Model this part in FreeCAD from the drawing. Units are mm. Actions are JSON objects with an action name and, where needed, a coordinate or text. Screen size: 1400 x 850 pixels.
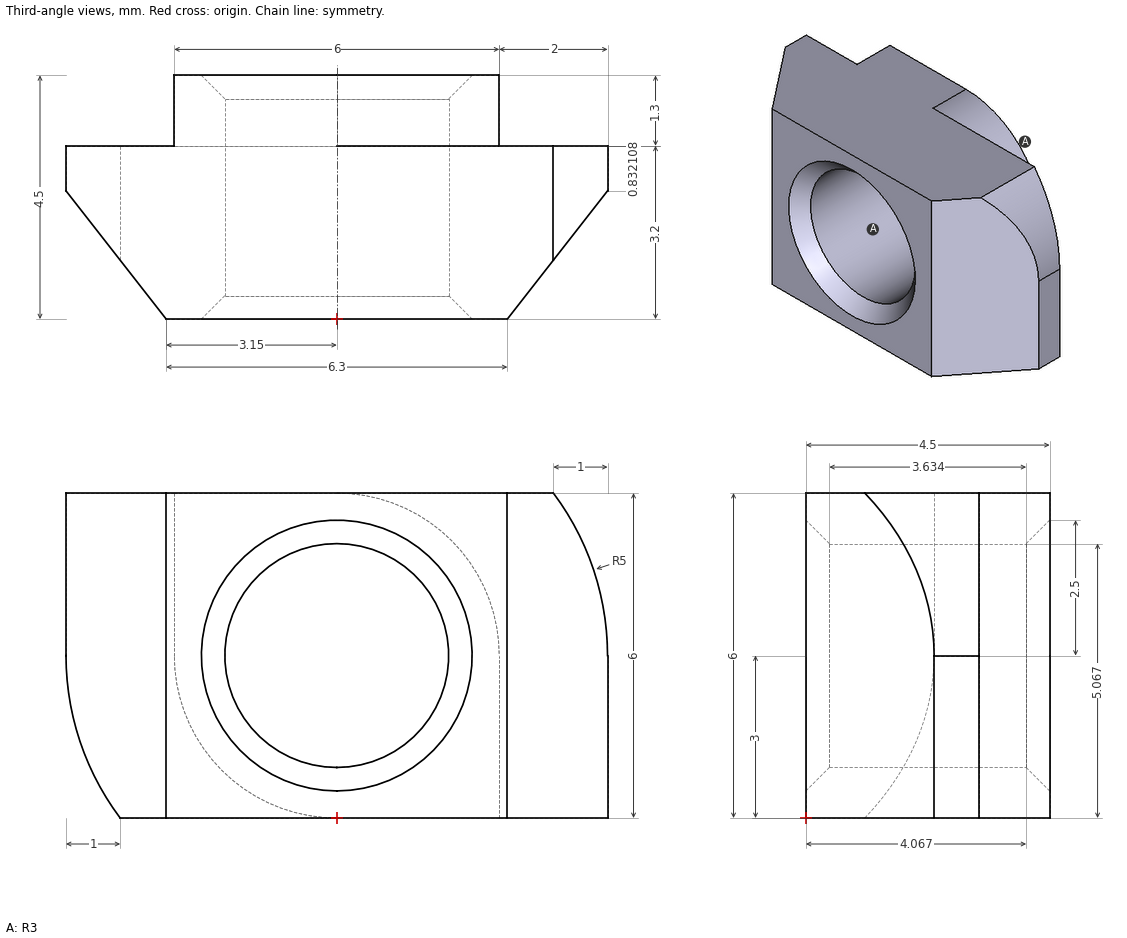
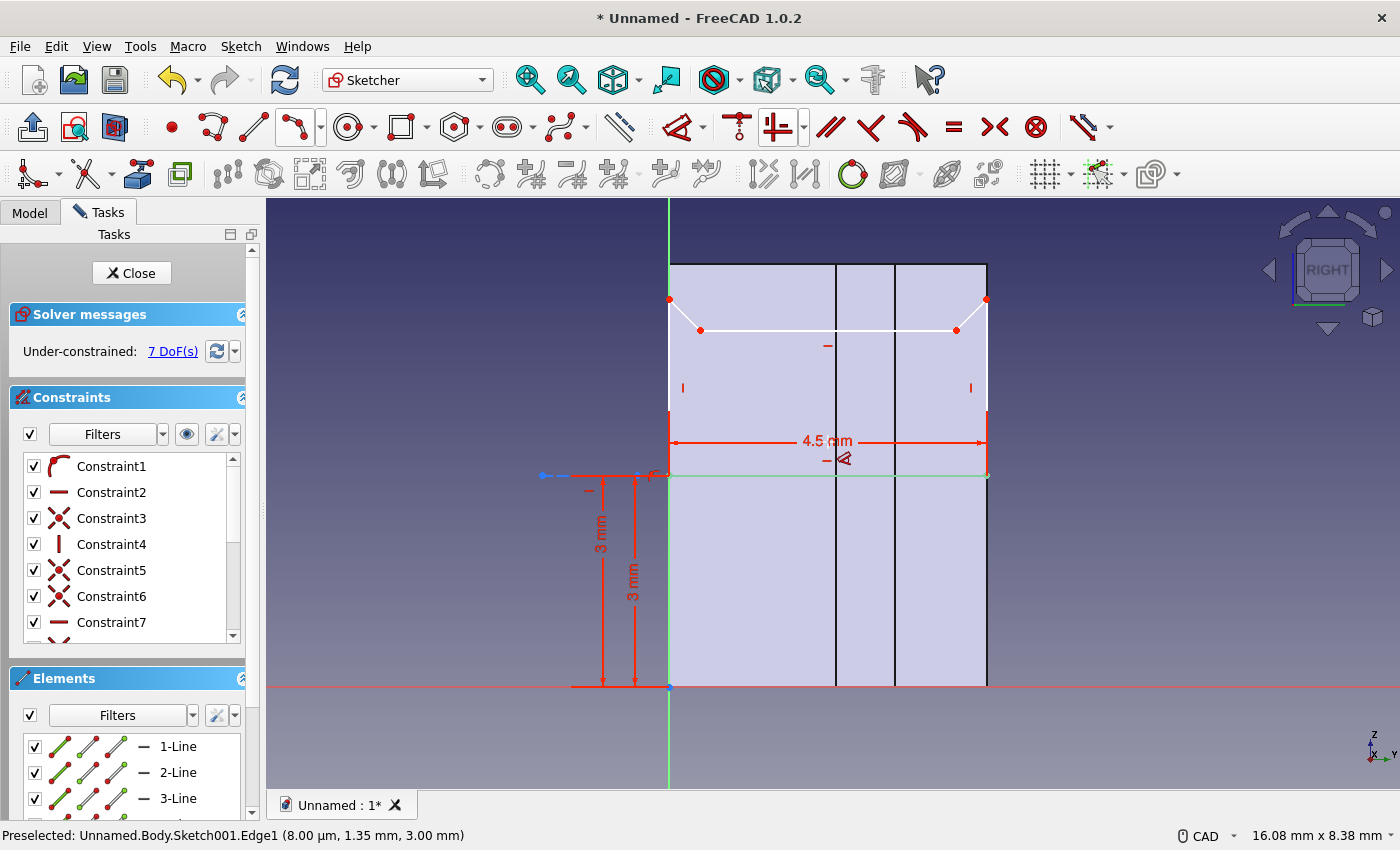
{"action": "left_click", "coordinate": [987, 423]}
{"action": "left_click", "coordinate": [1021, 388]}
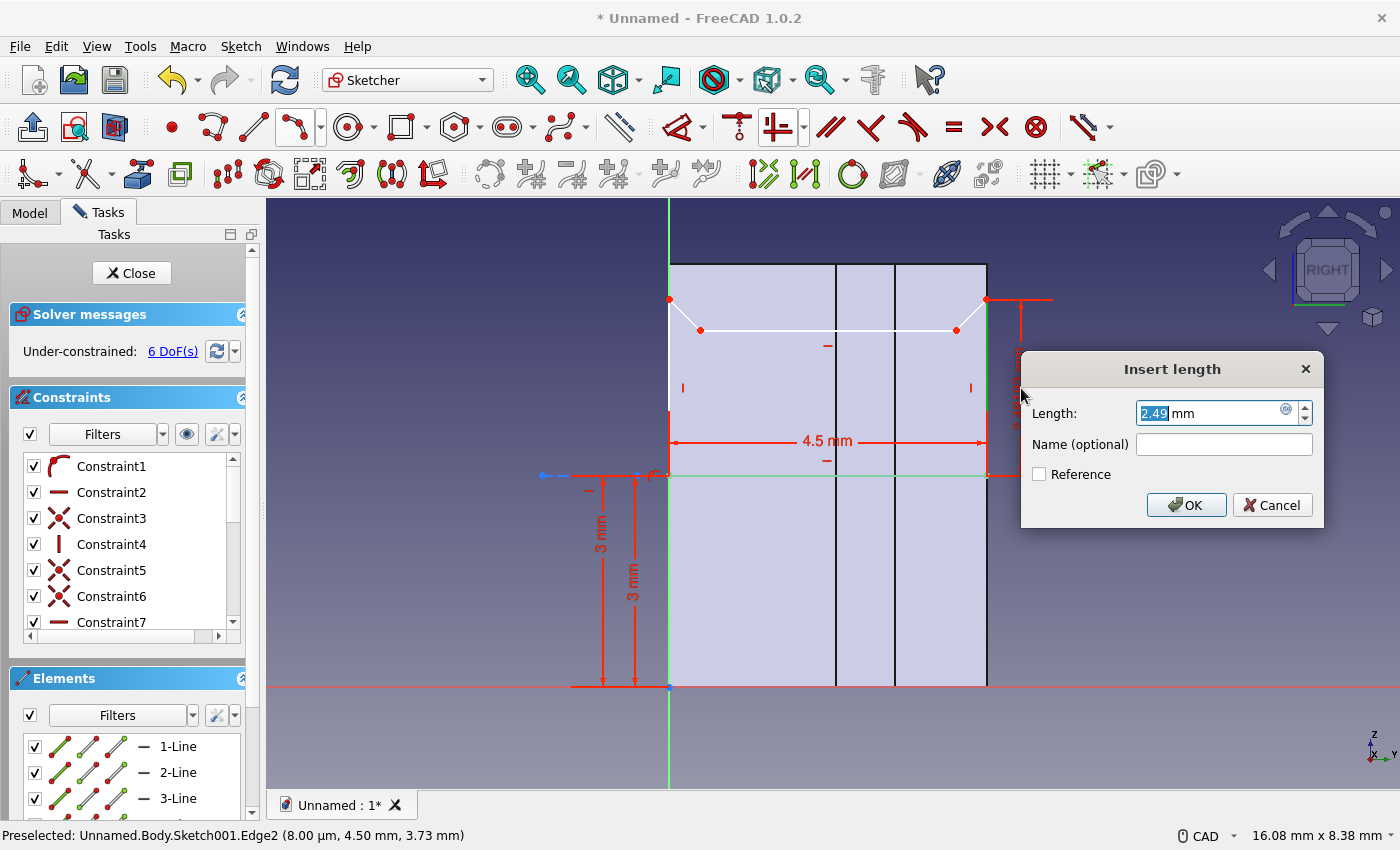
{"action": "type", "text": "2.5"}
{"action": "key", "text": "Return"}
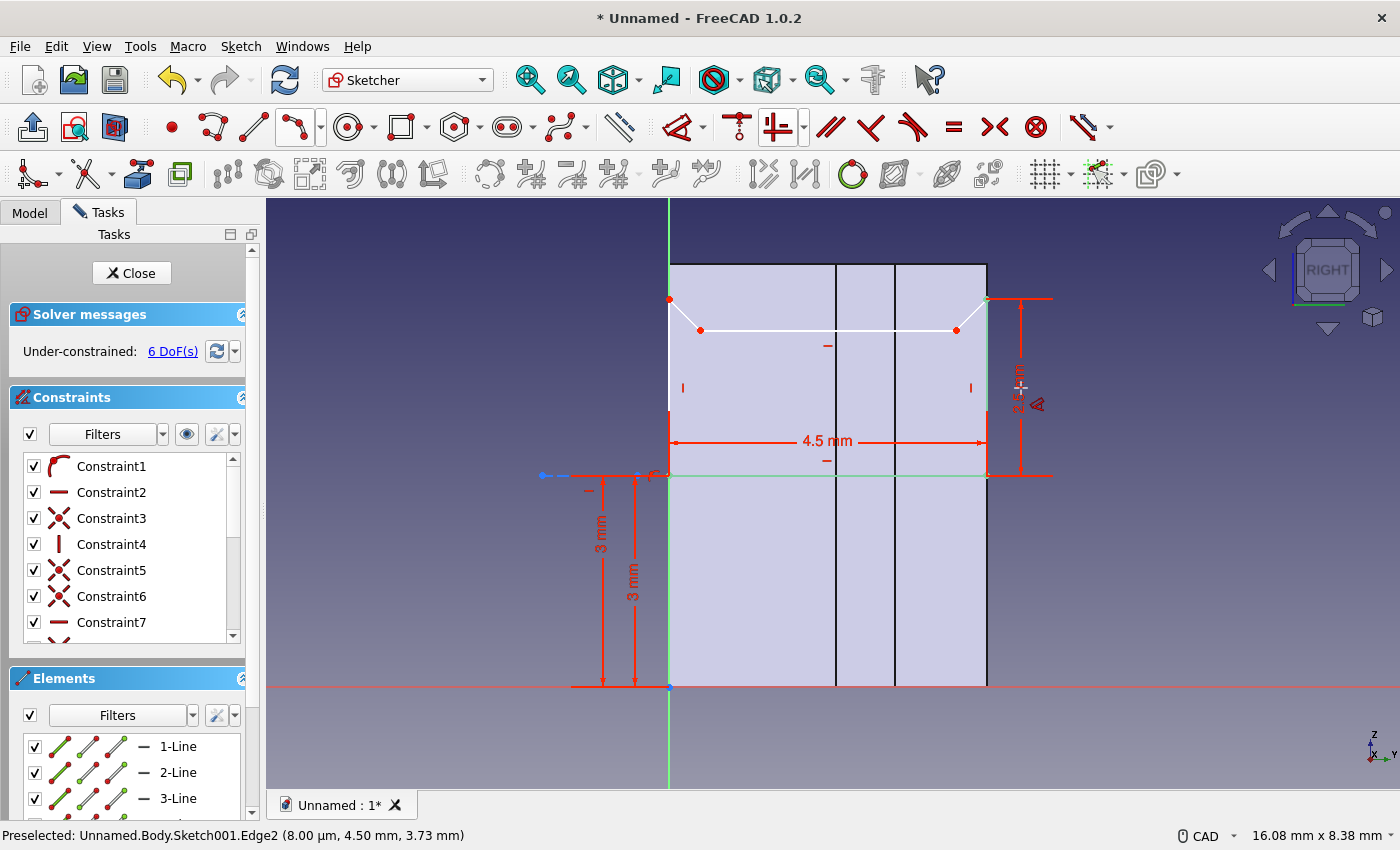
{"action": "left_click", "coordinate": [669, 353]}
{"action": "left_click", "coordinate": [635, 388]}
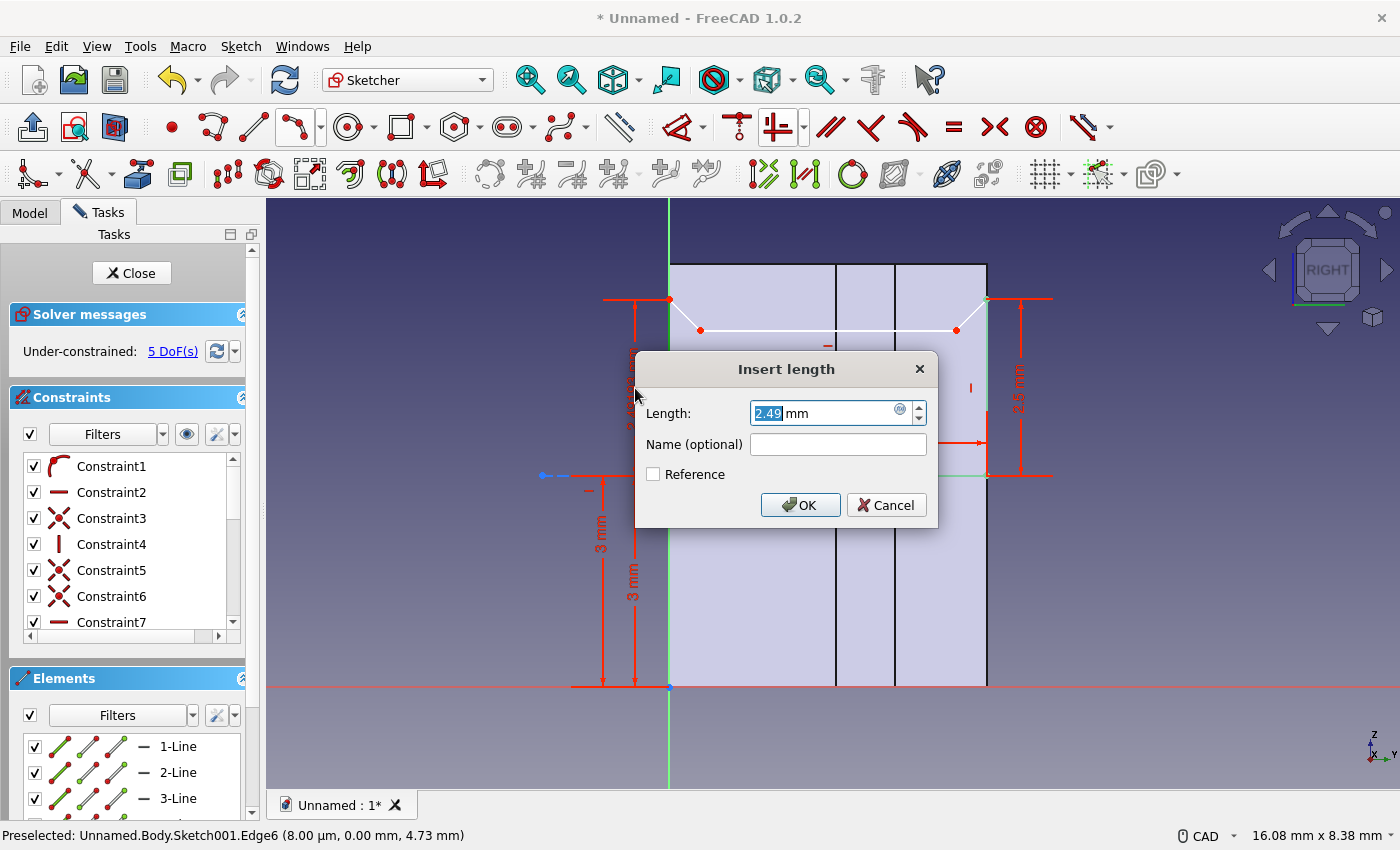
{"action": "type", "text": "2.5"}
{"action": "key", "text": "Return"}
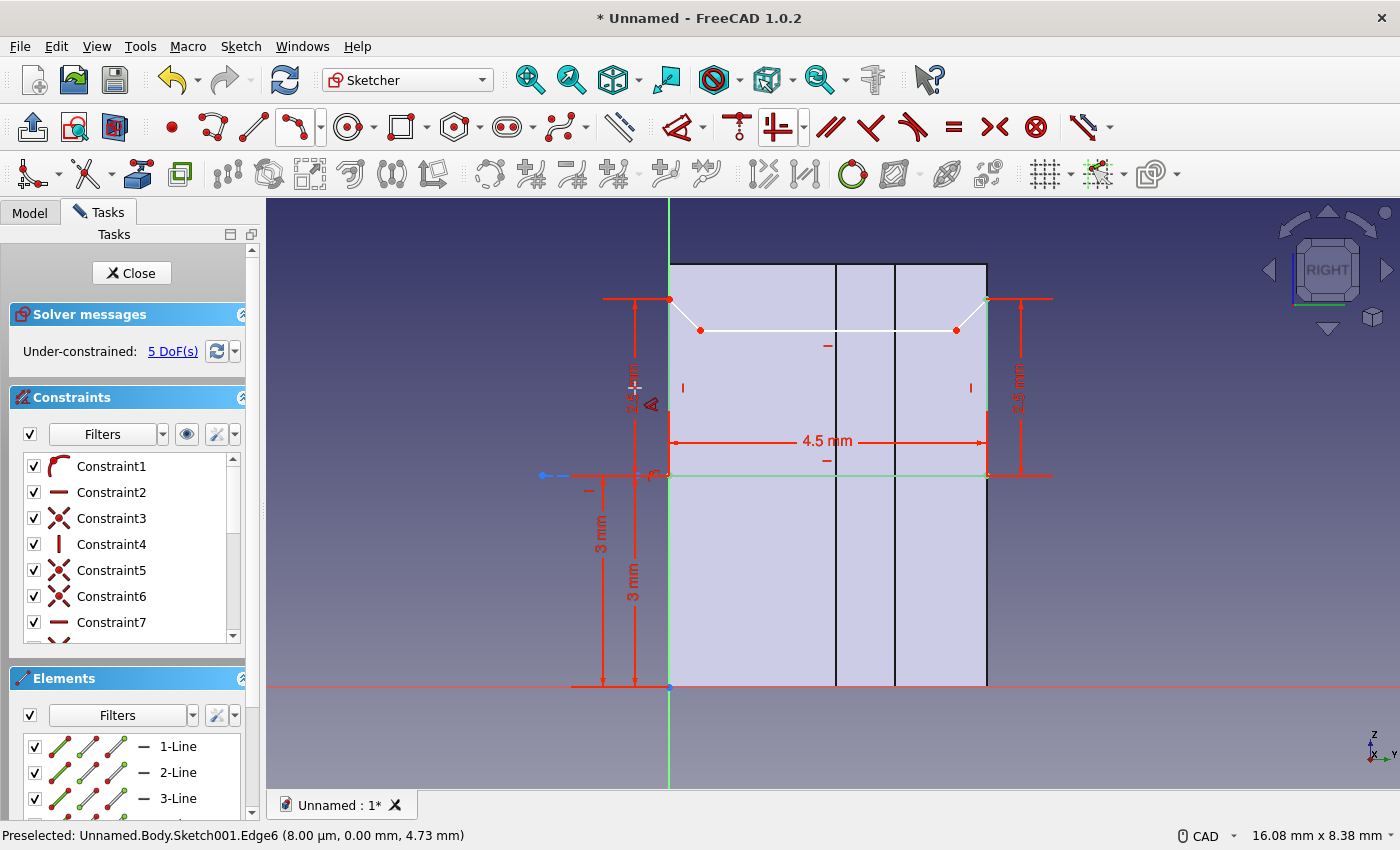
{"action": "left_click", "coordinate": [879, 331]}
{"action": "left_click", "coordinate": [828, 297]}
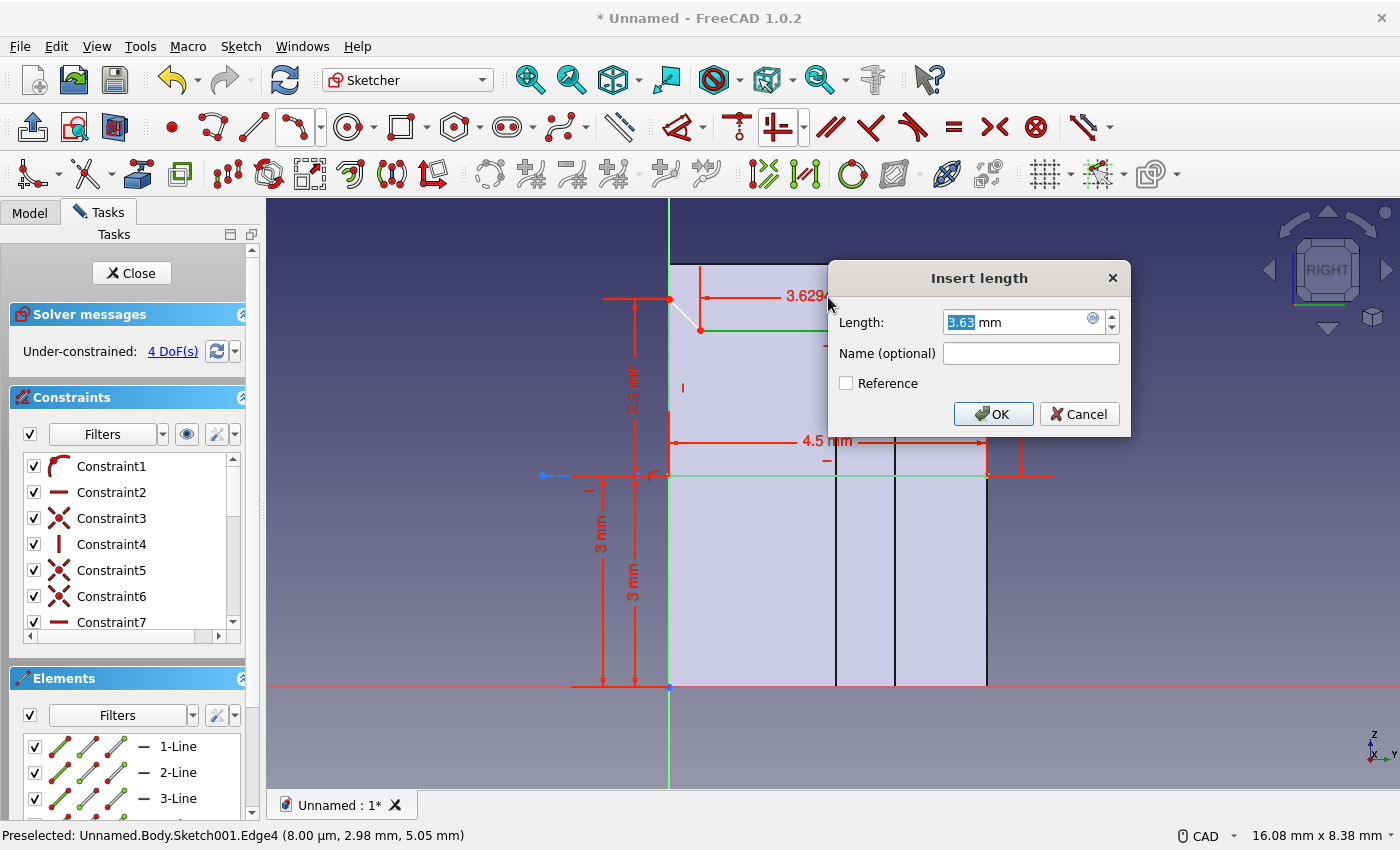
{"action": "type", "text": "3.634"}
{"action": "key", "text": "Return"}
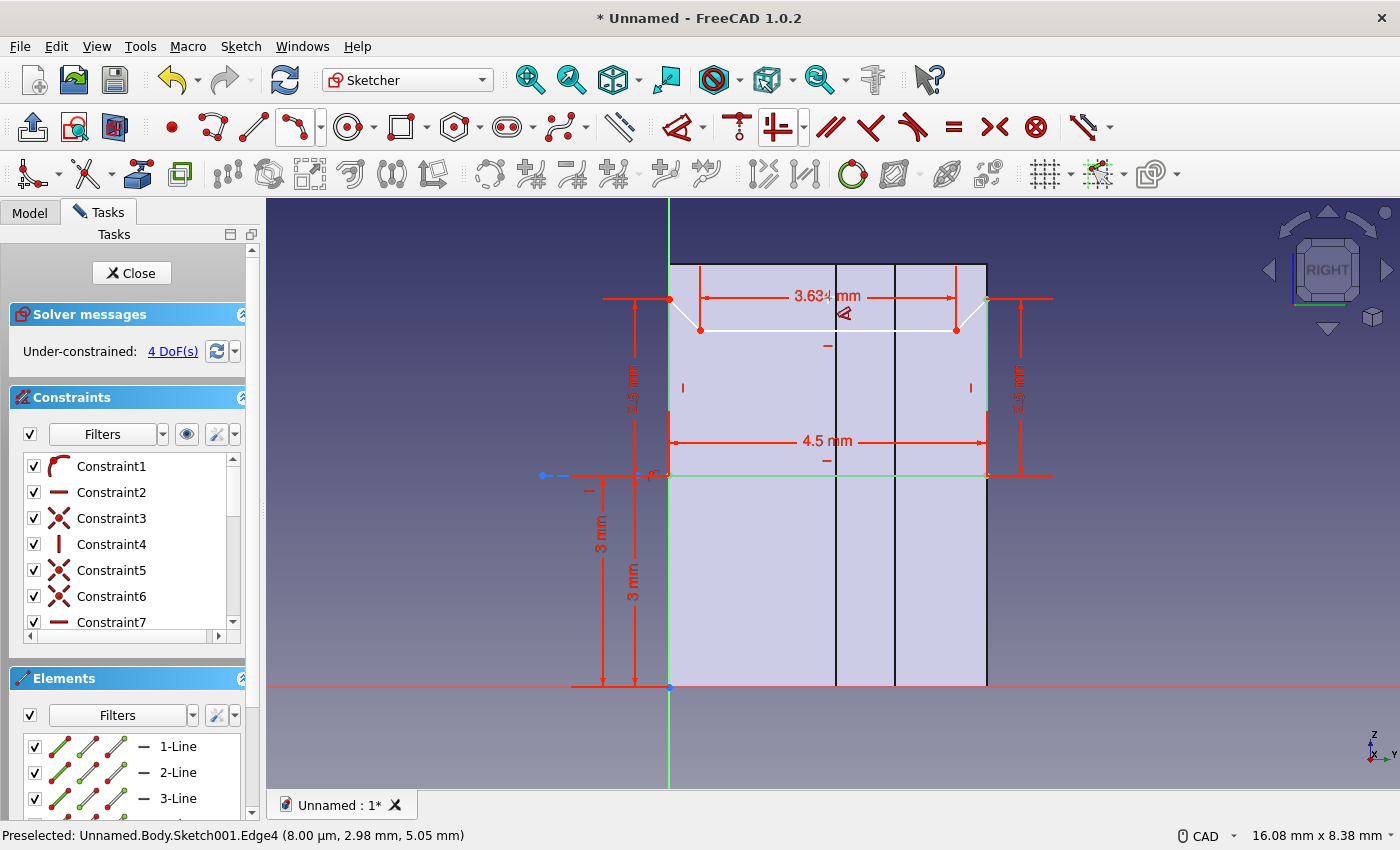
{"action": "left_click", "coordinate": [956, 331]}
{"action": "left_click", "coordinate": [813, 721]}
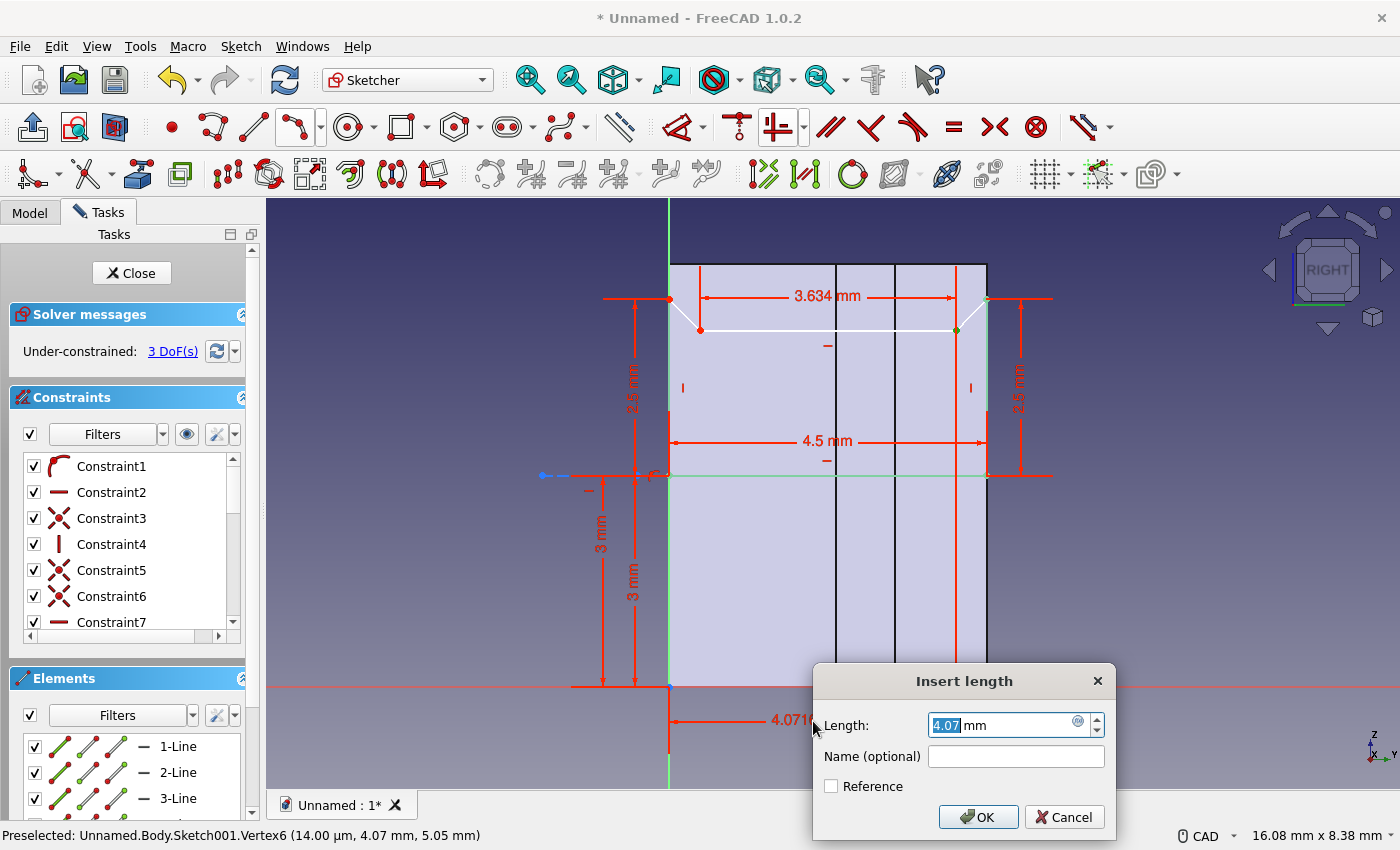
{"action": "type", "text": "4.067"}
{"action": "key", "text": "Return"}